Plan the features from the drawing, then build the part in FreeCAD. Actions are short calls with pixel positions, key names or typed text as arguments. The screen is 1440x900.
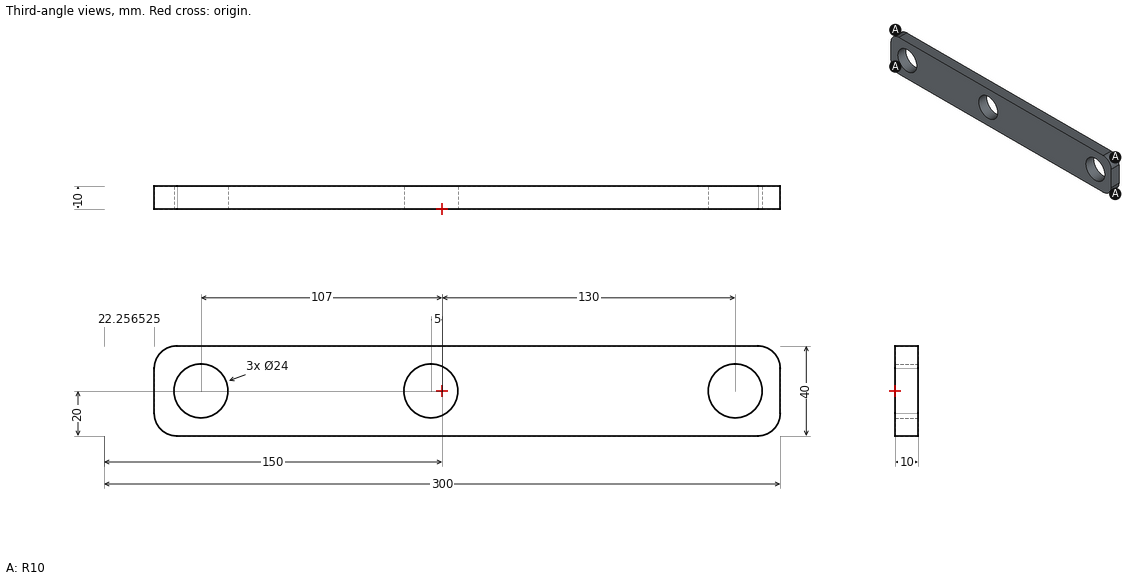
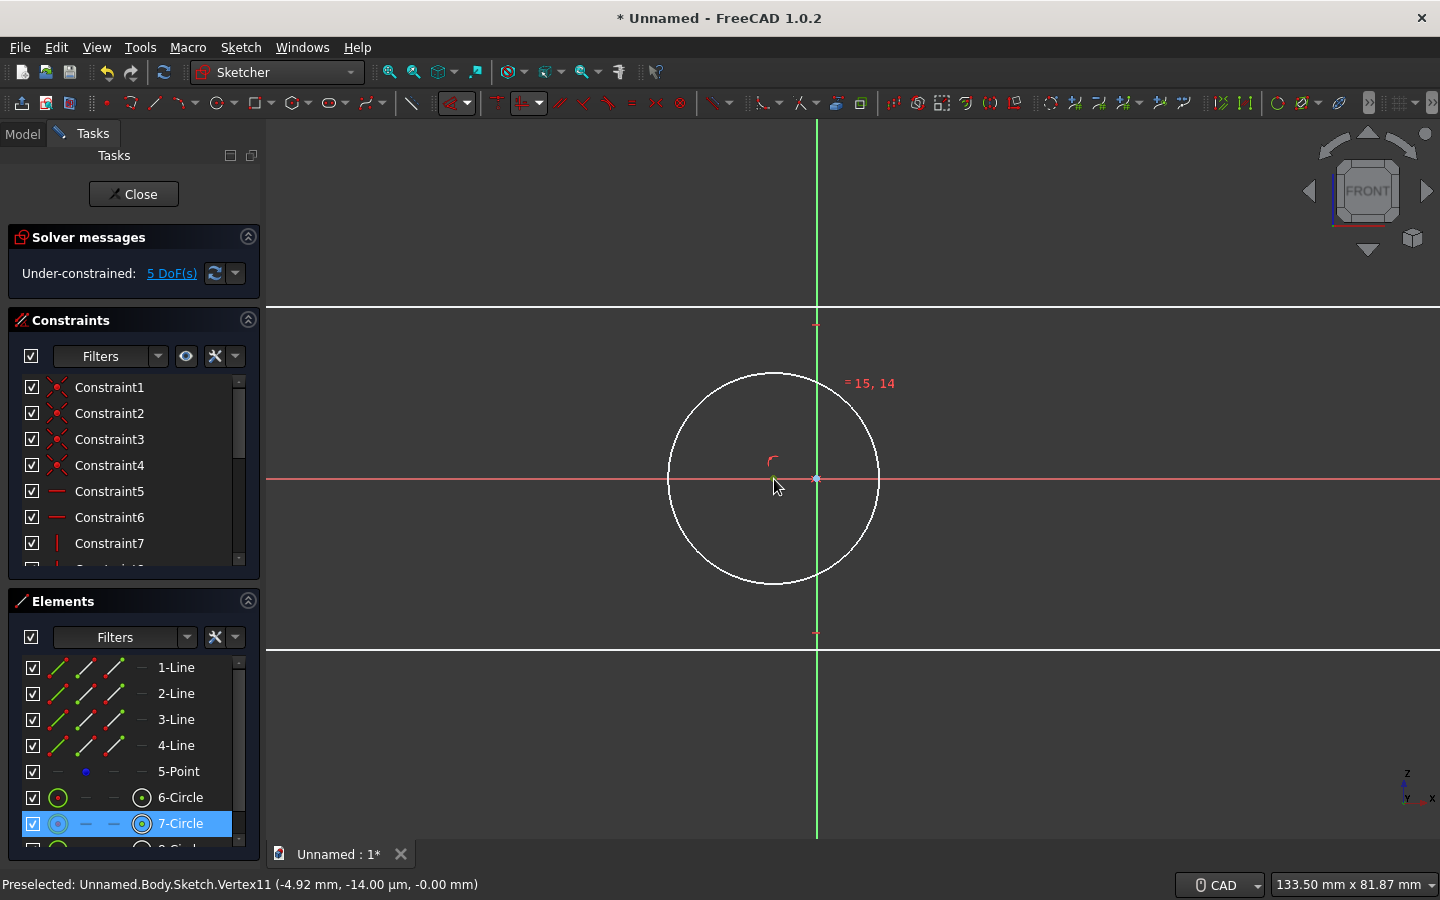
key(l)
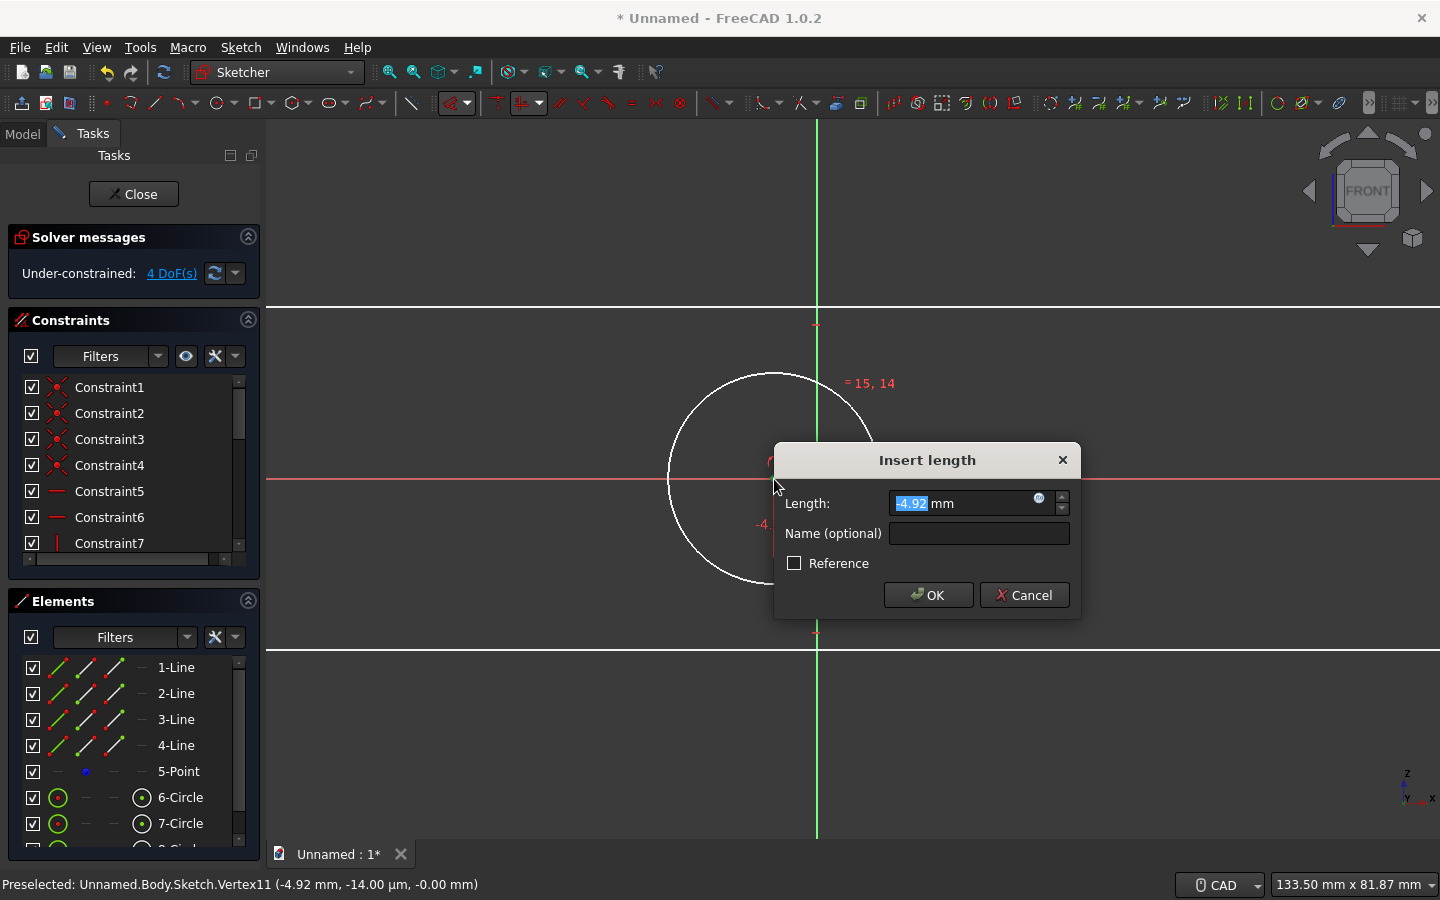
text(-5)
key(Return)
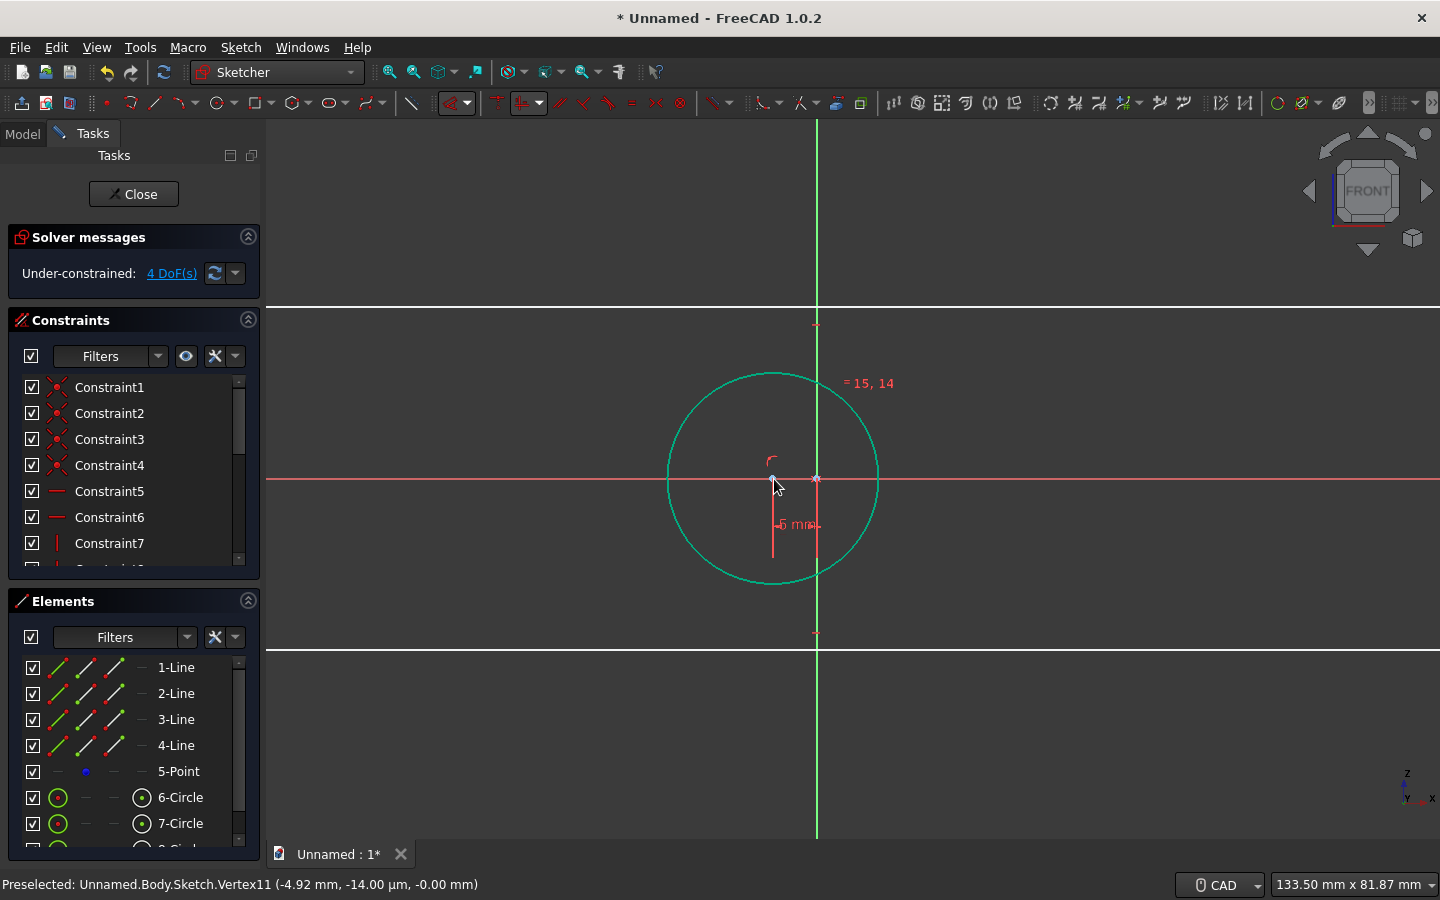
scroll(774, 479, down, 7)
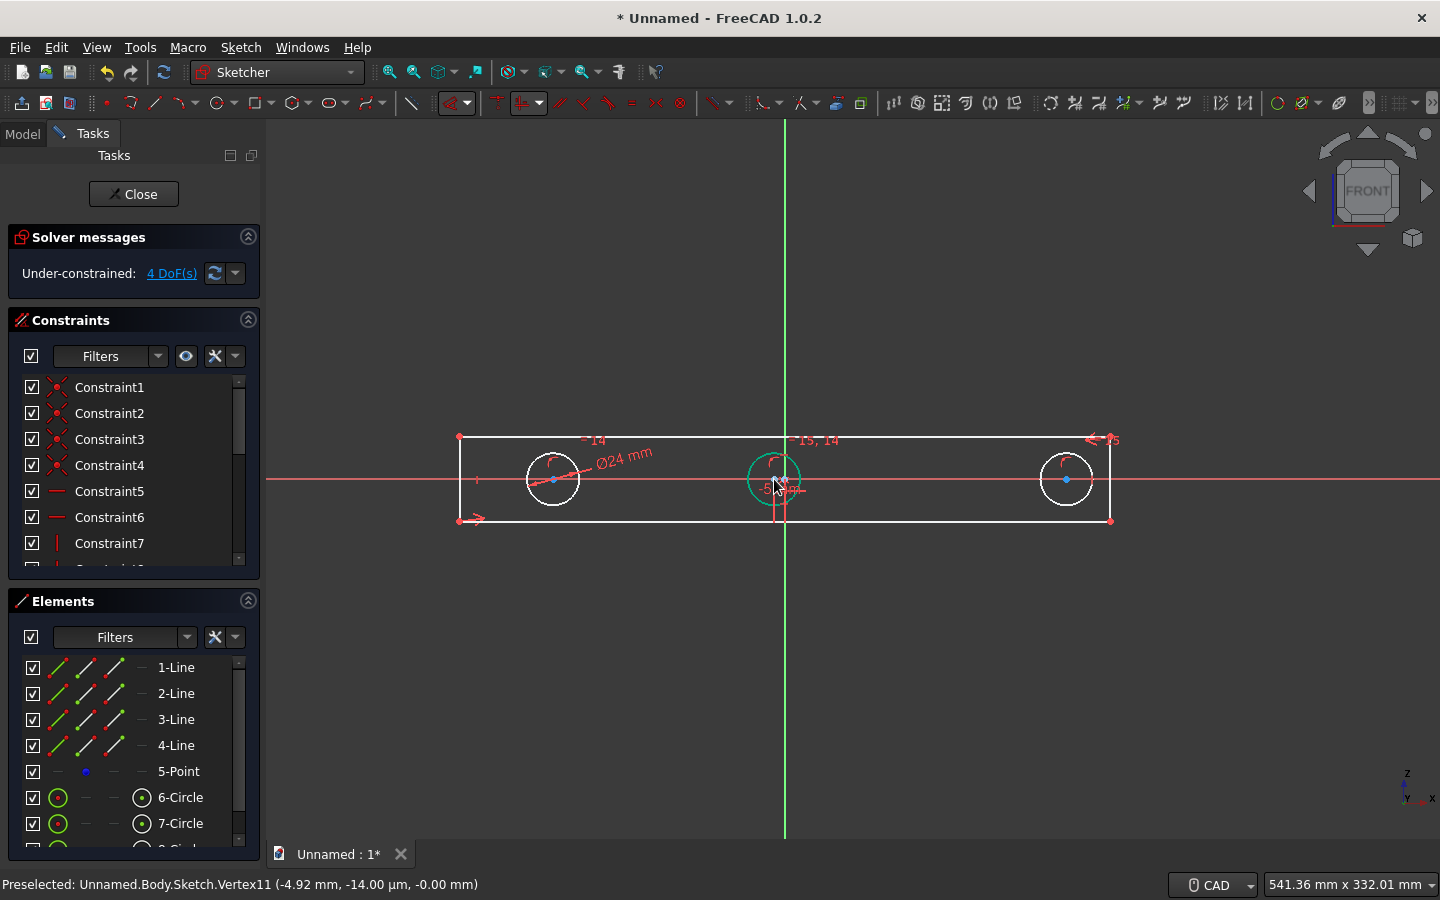
click(1110, 496)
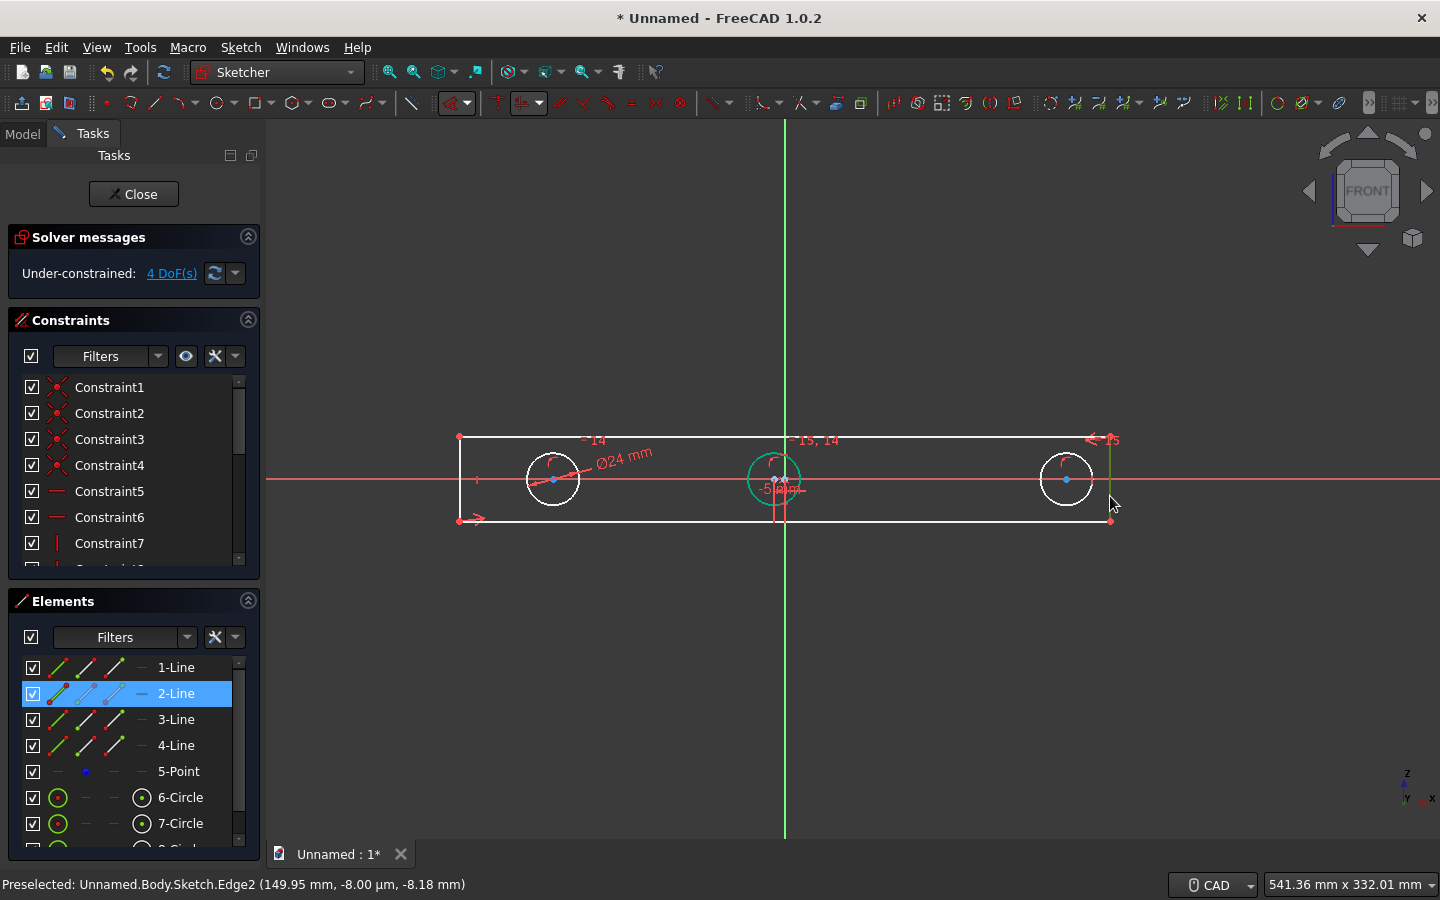
click(470, 104)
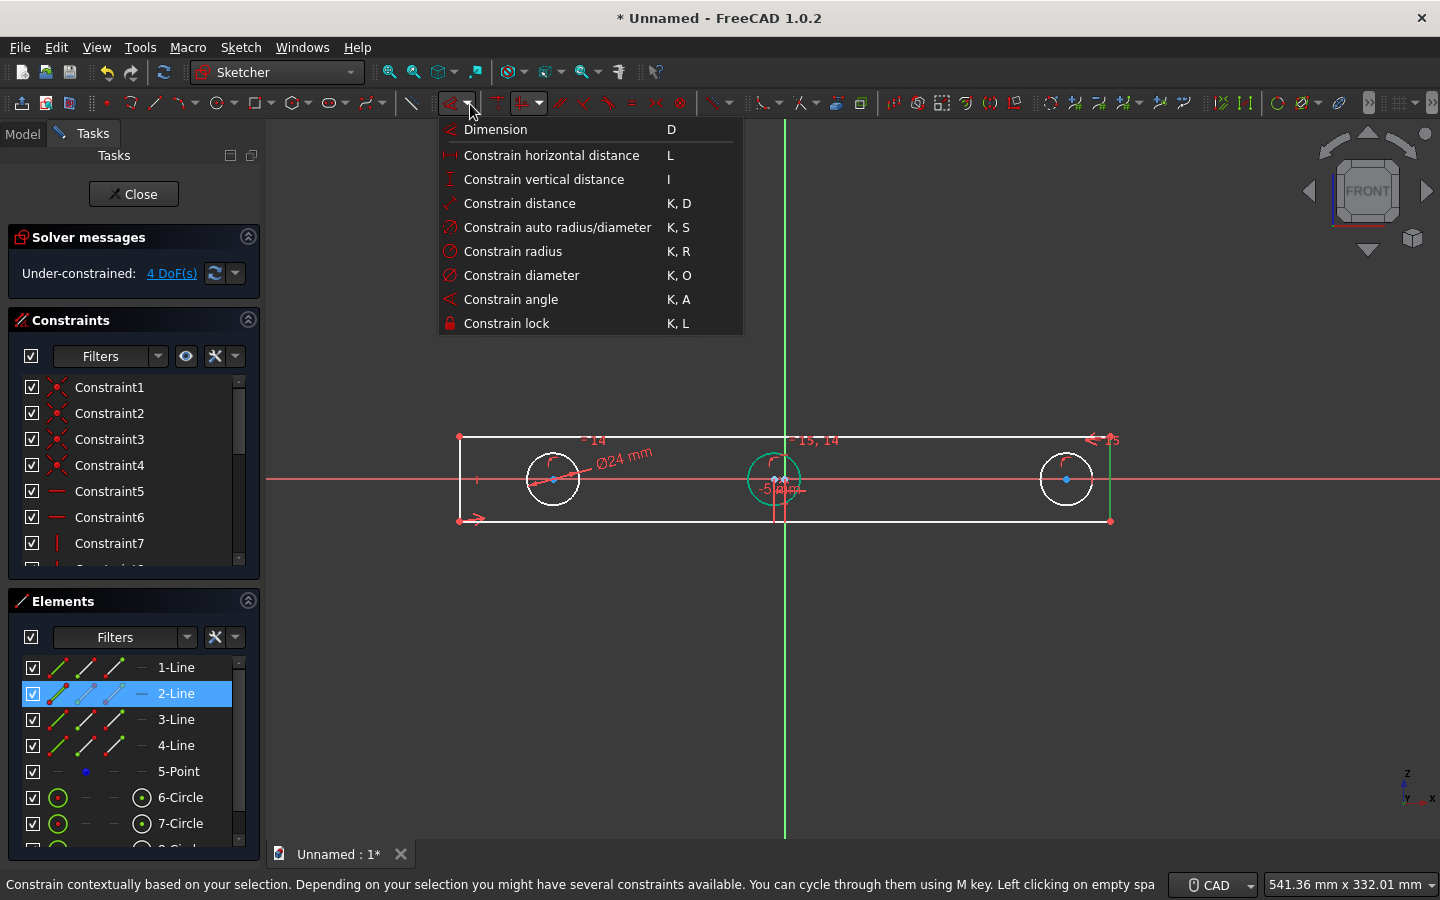
click(591, 179)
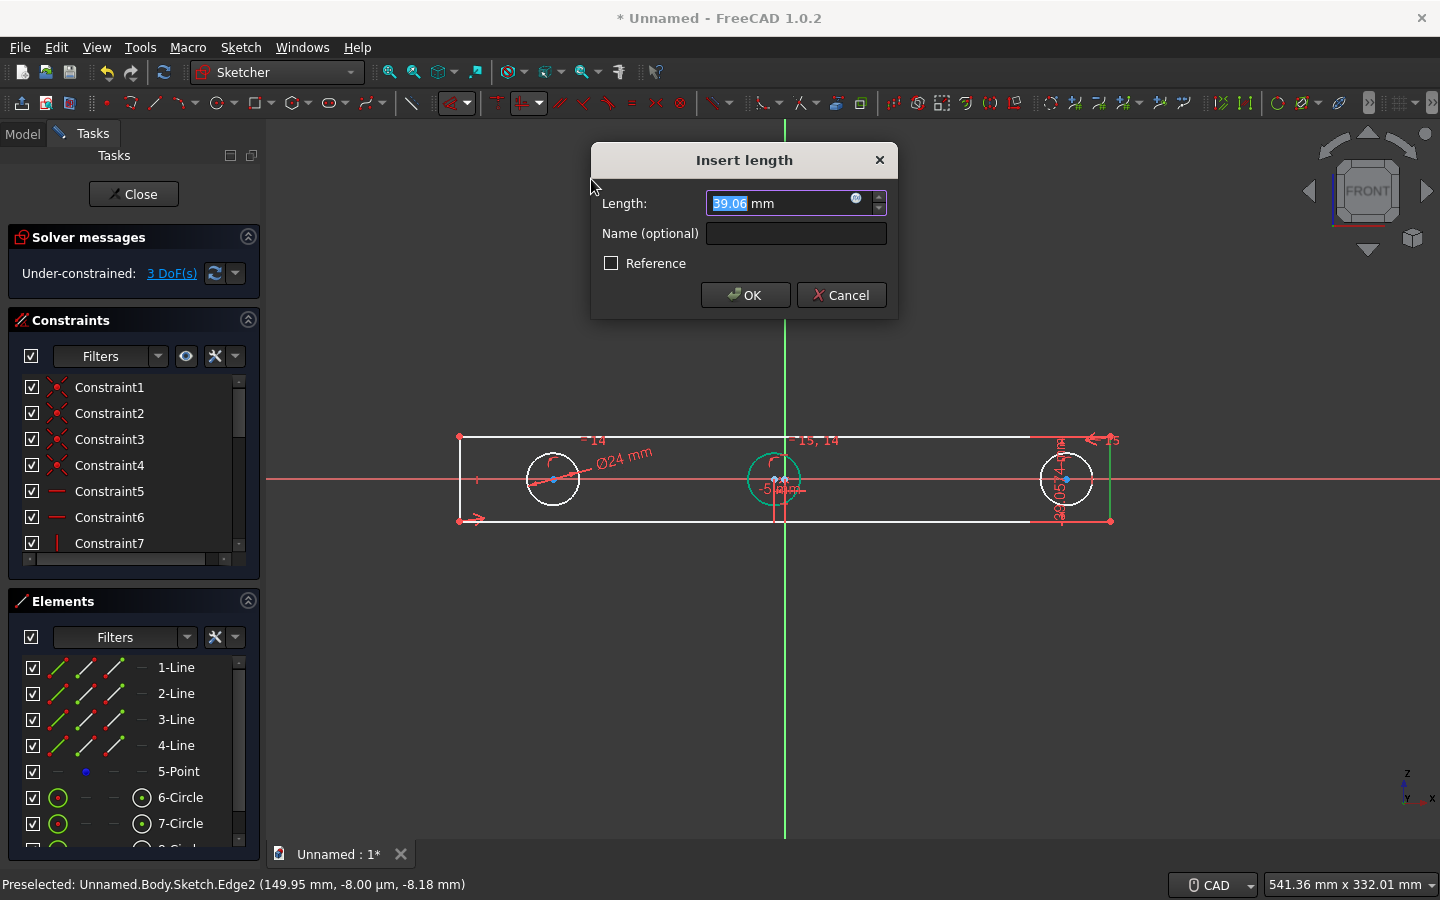
text(40)
key(Return)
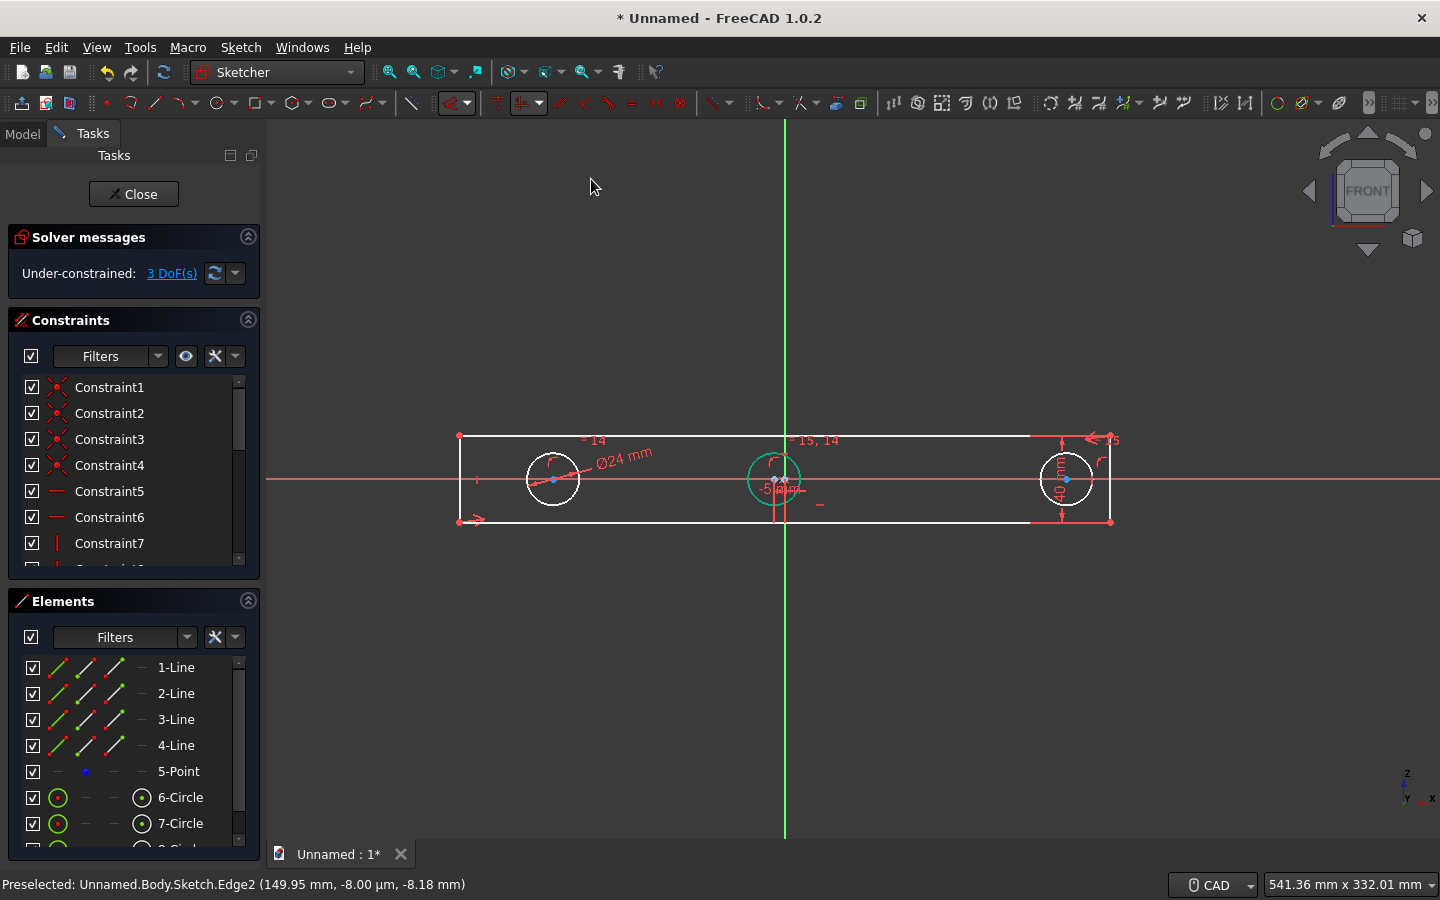
click(655, 523)